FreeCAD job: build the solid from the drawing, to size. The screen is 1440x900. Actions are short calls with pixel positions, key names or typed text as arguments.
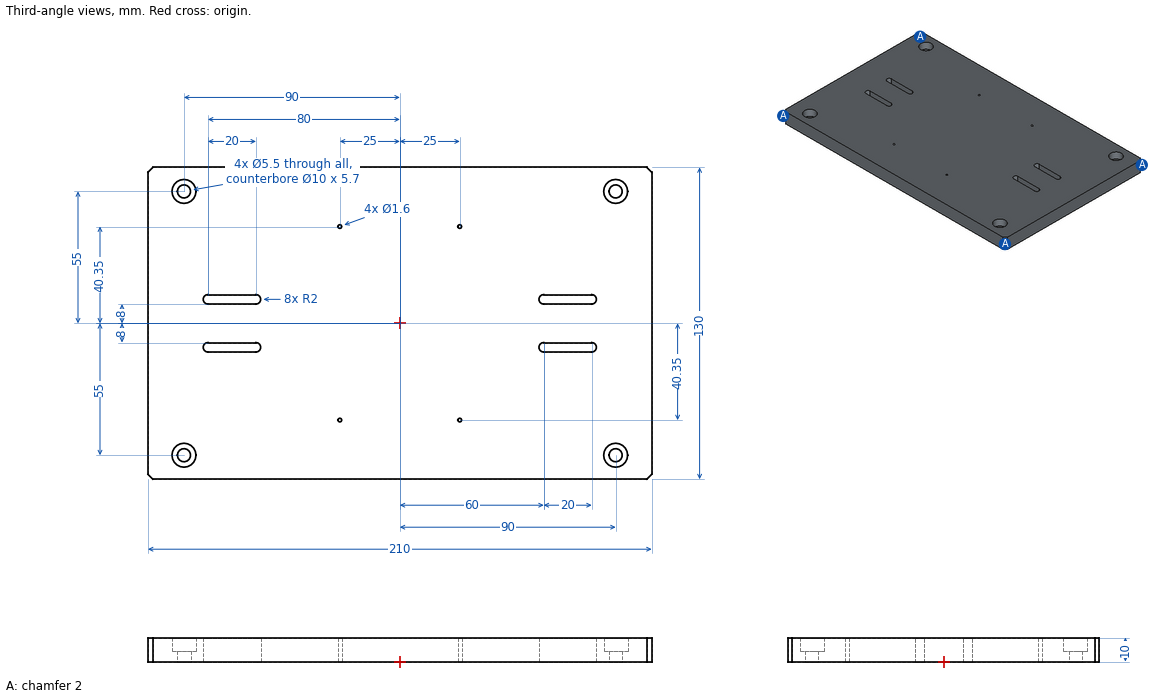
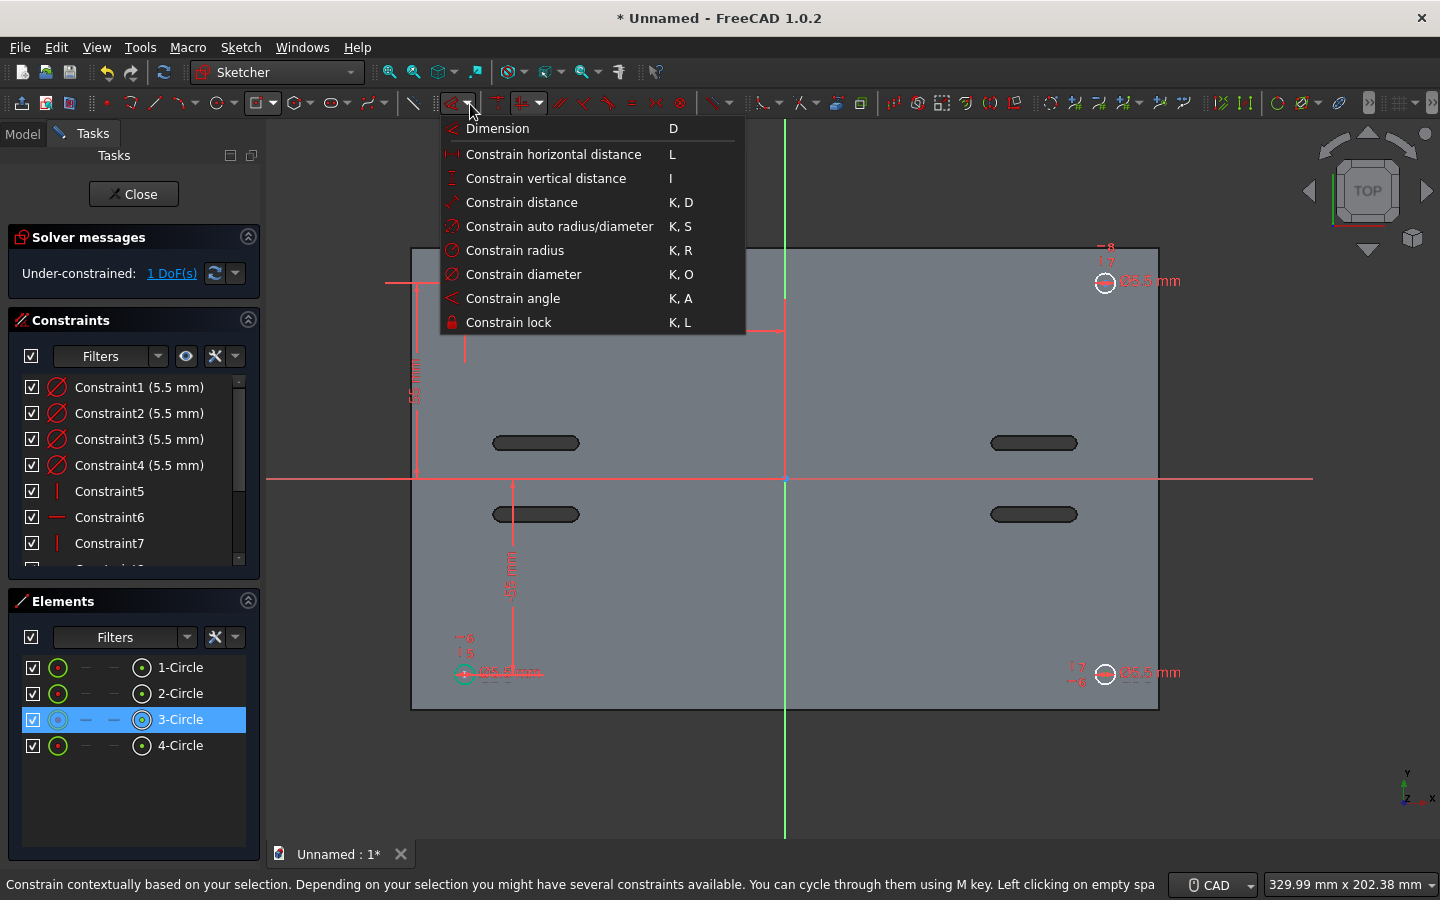
click(593, 154)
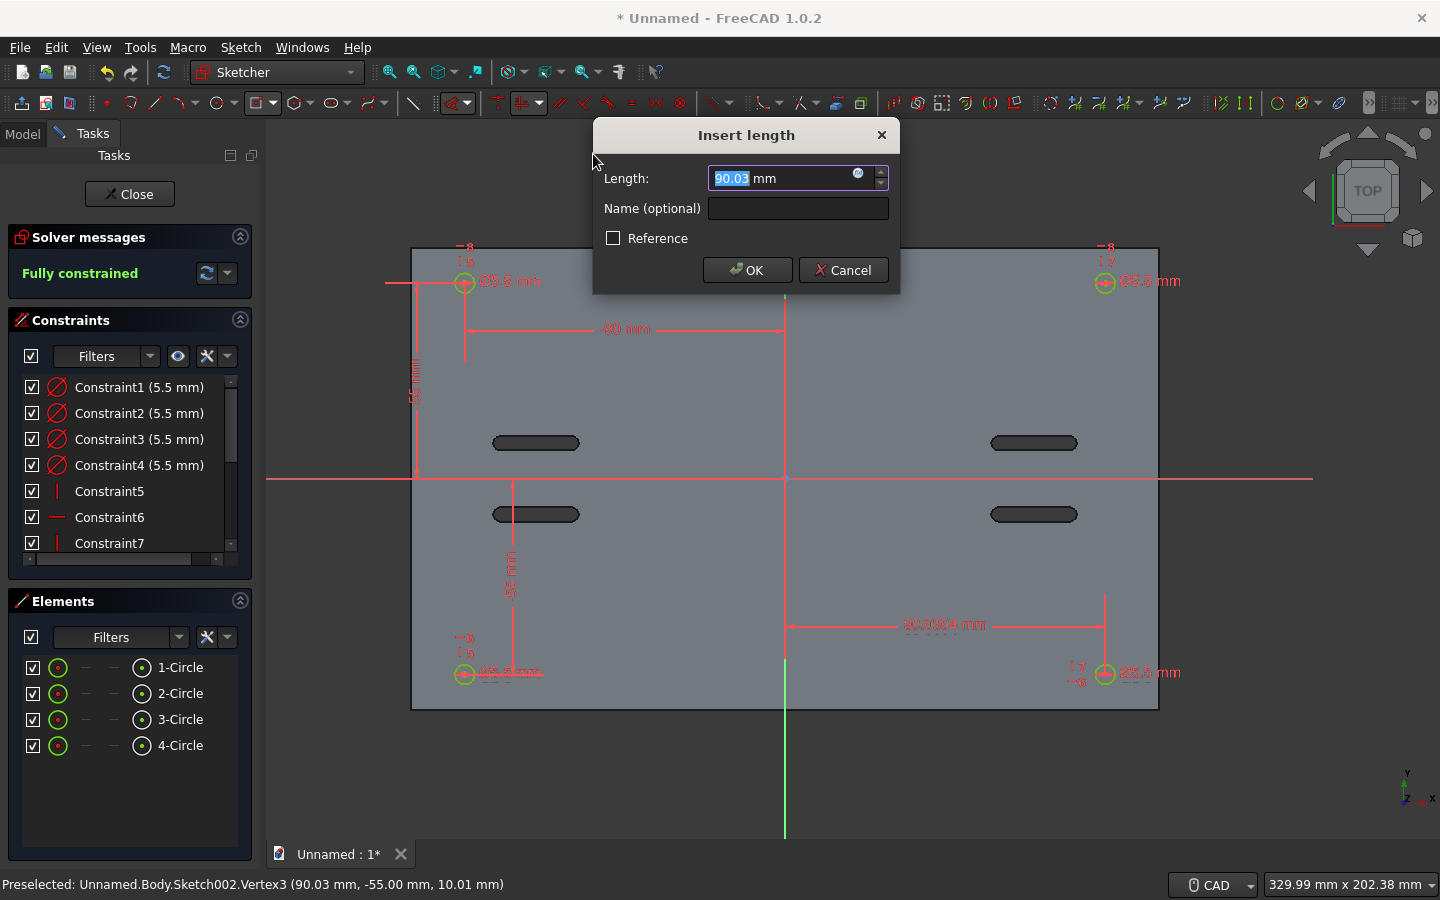
text(90)
key(Return)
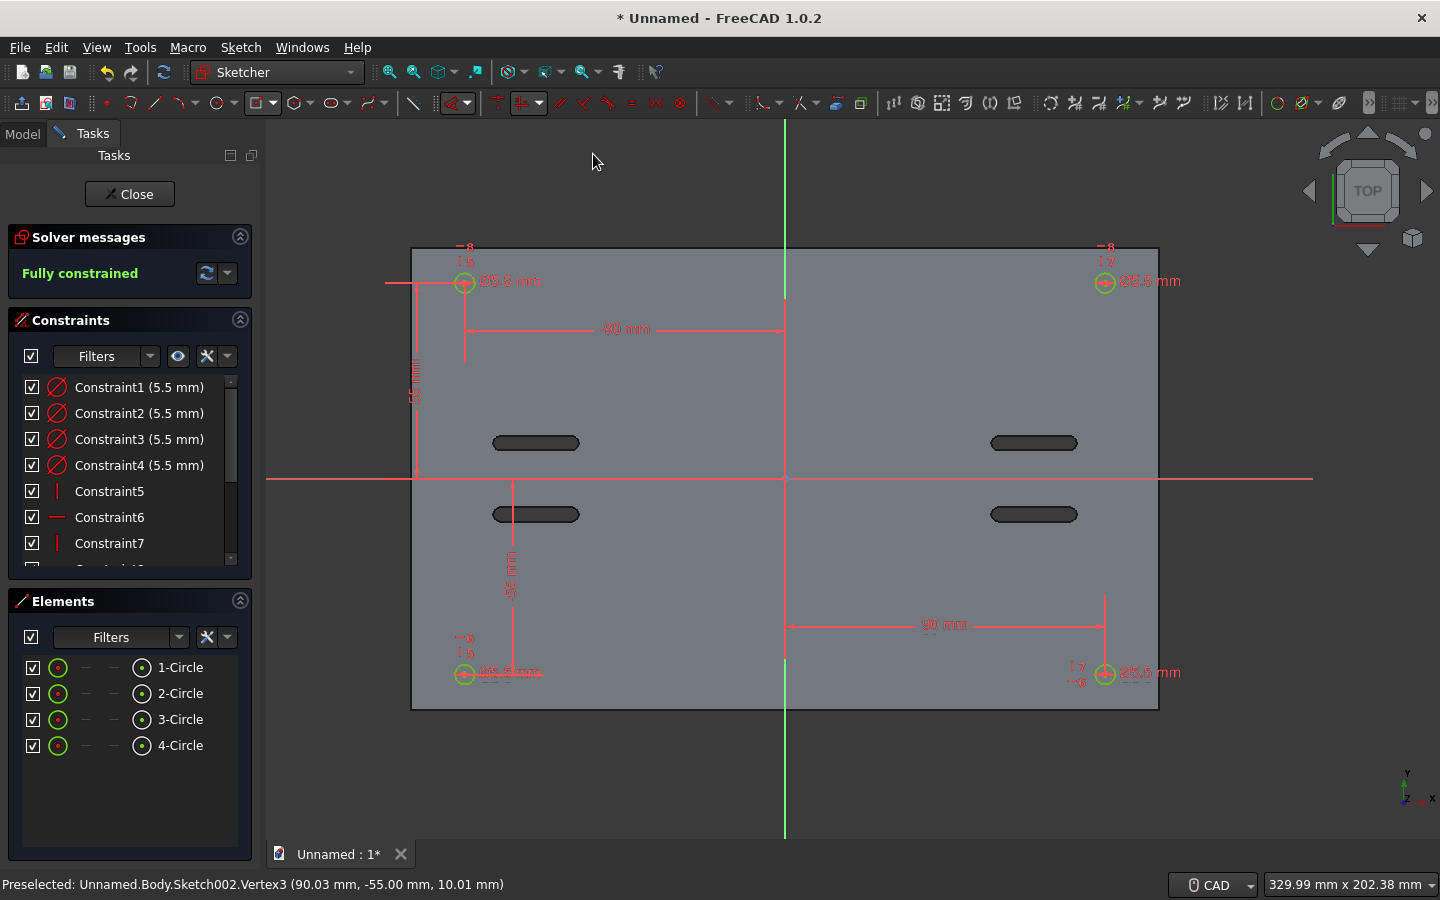
click(130, 194)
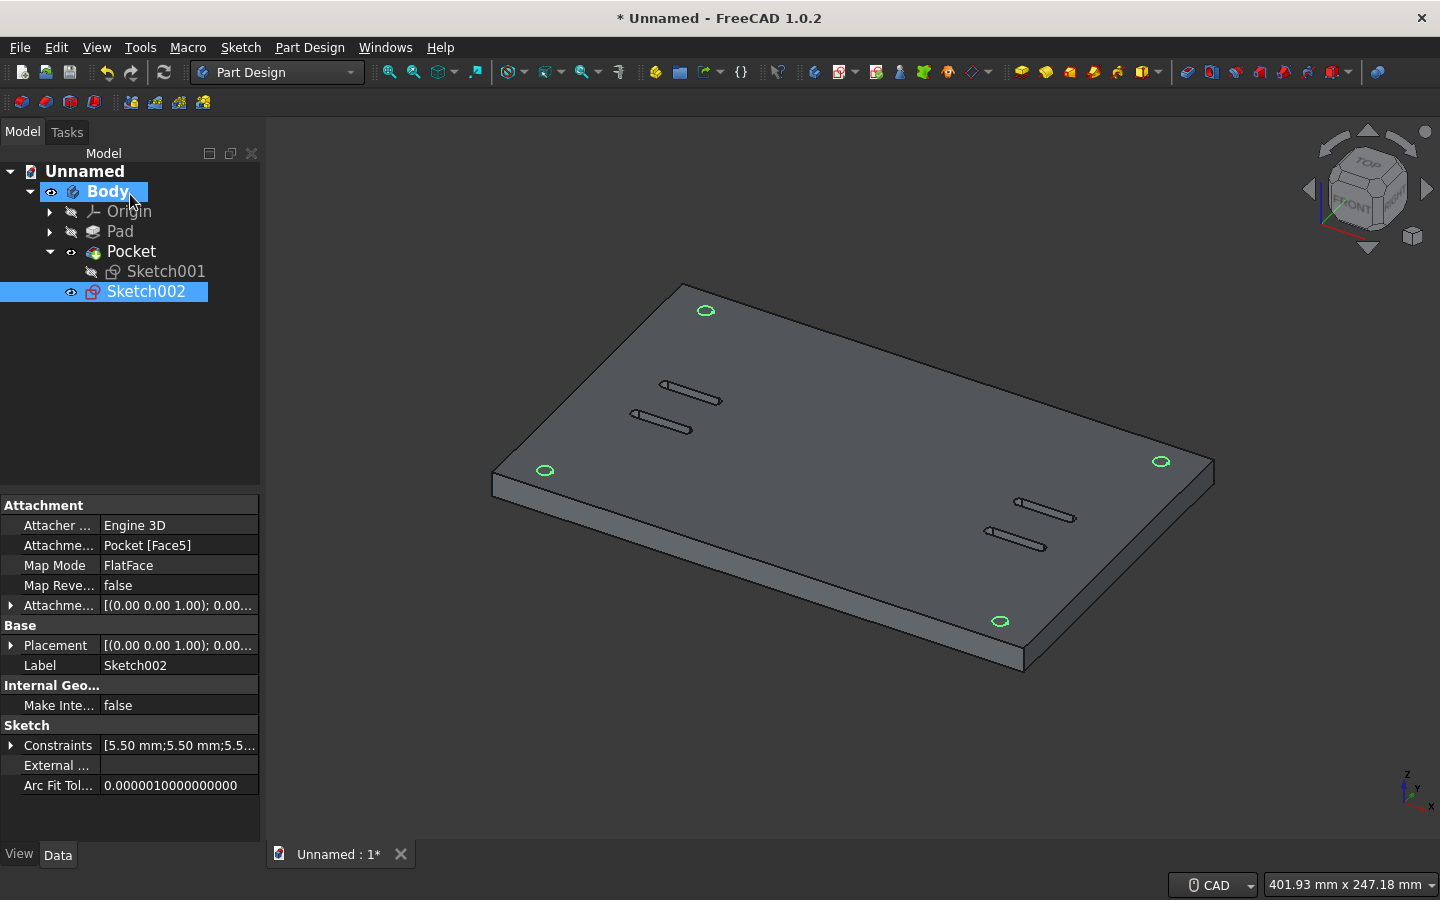
click(1212, 72)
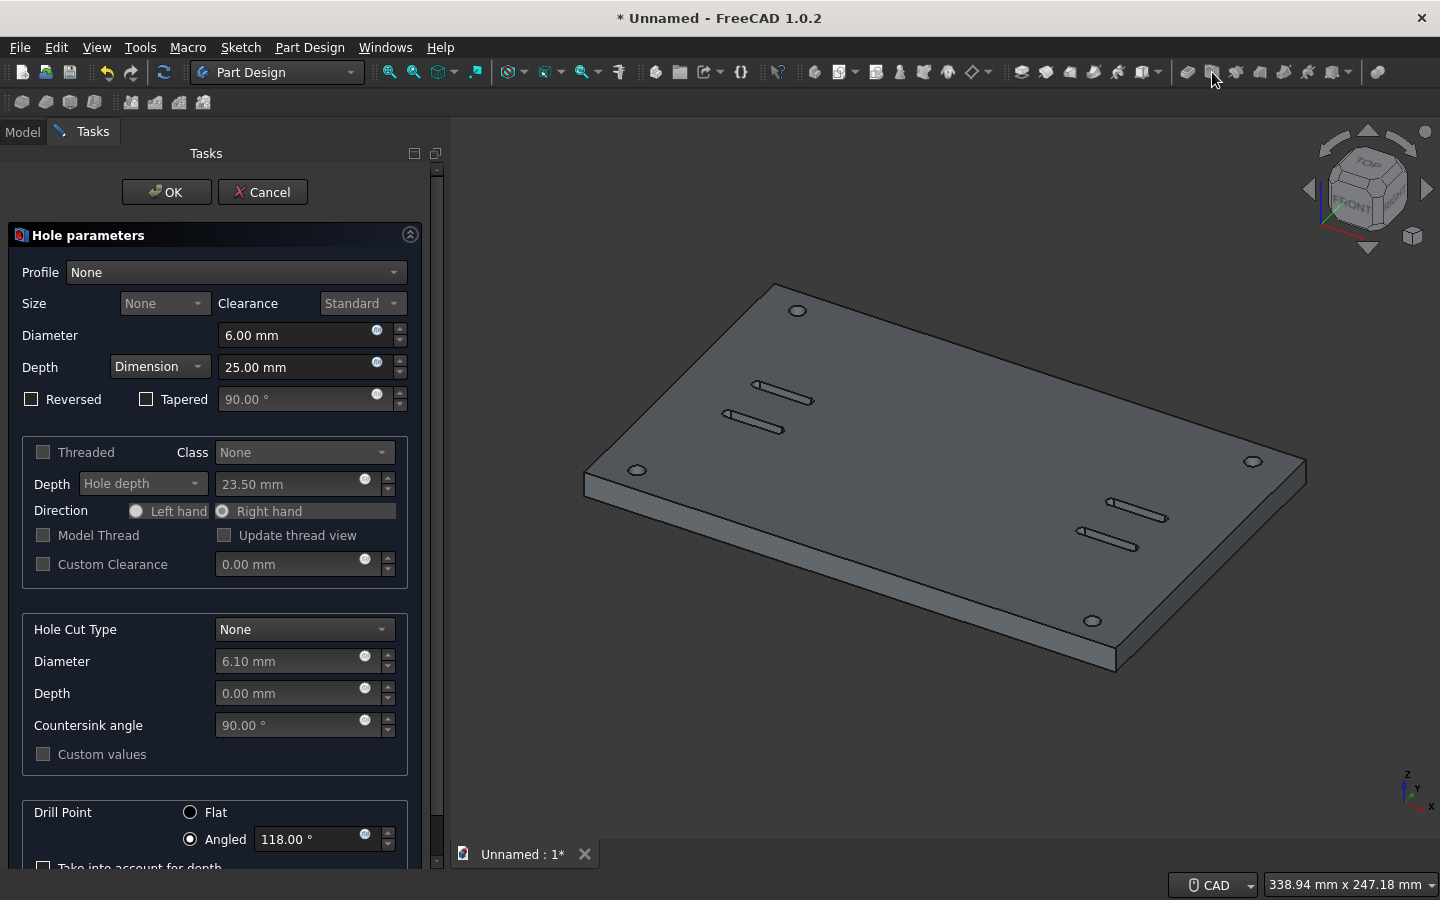
triple_click(305, 335)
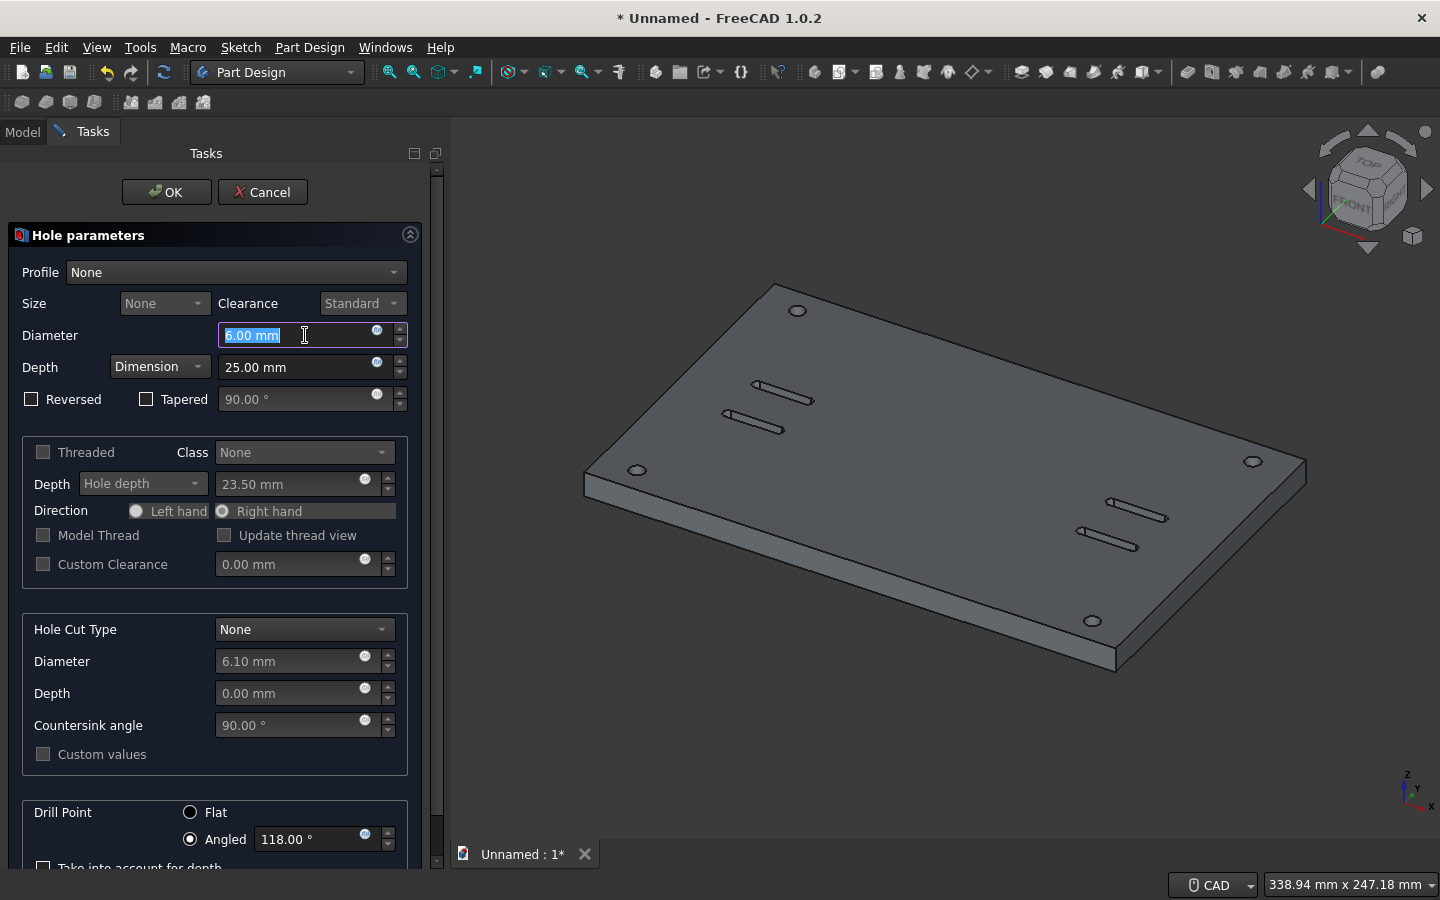
text(5.5)
key(Tab)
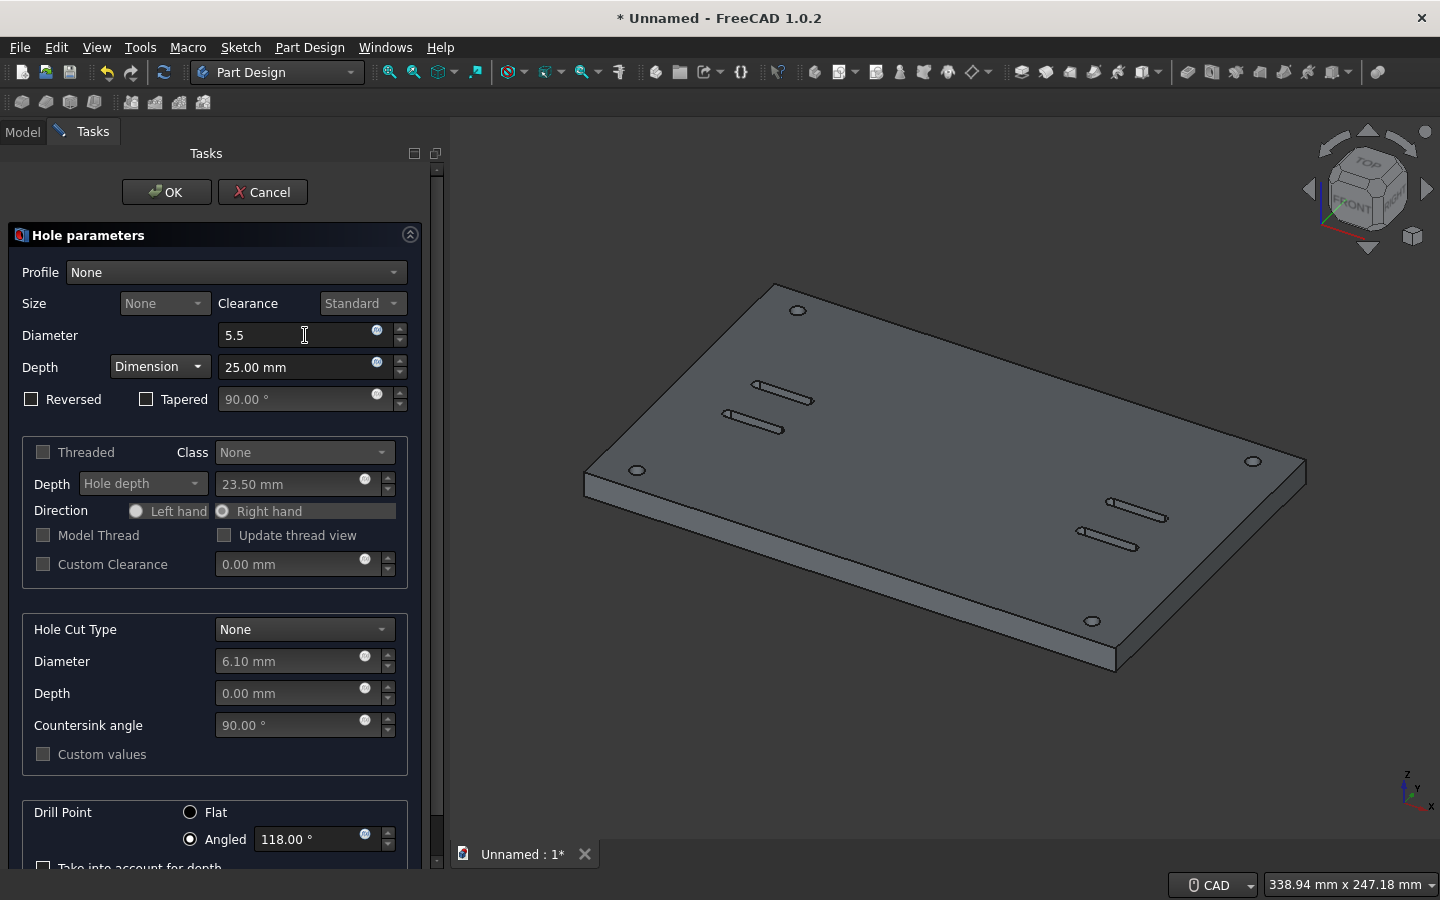
click(161, 366)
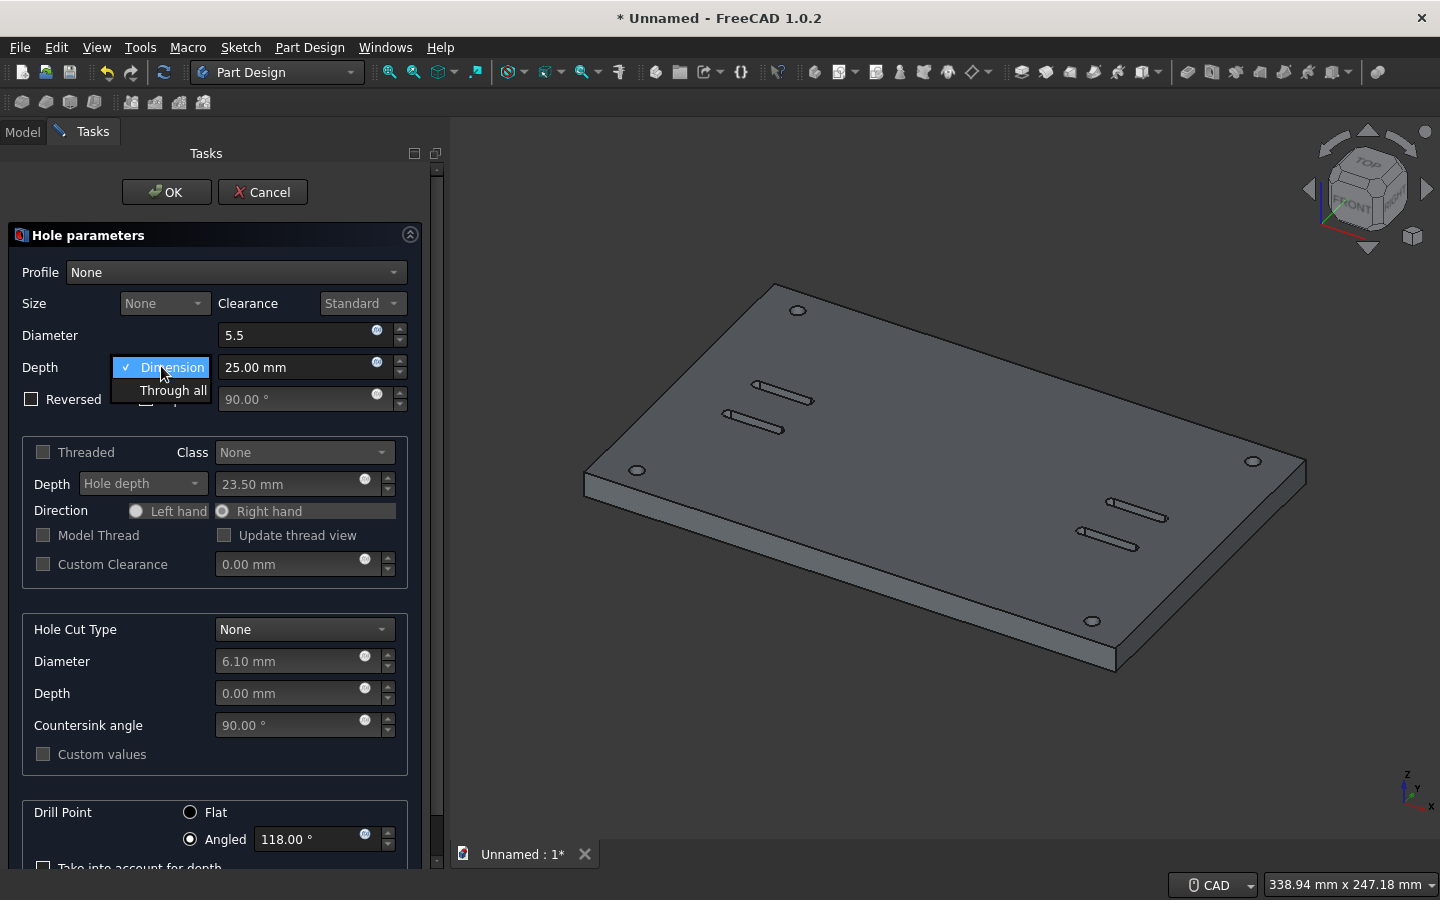
click(160, 390)